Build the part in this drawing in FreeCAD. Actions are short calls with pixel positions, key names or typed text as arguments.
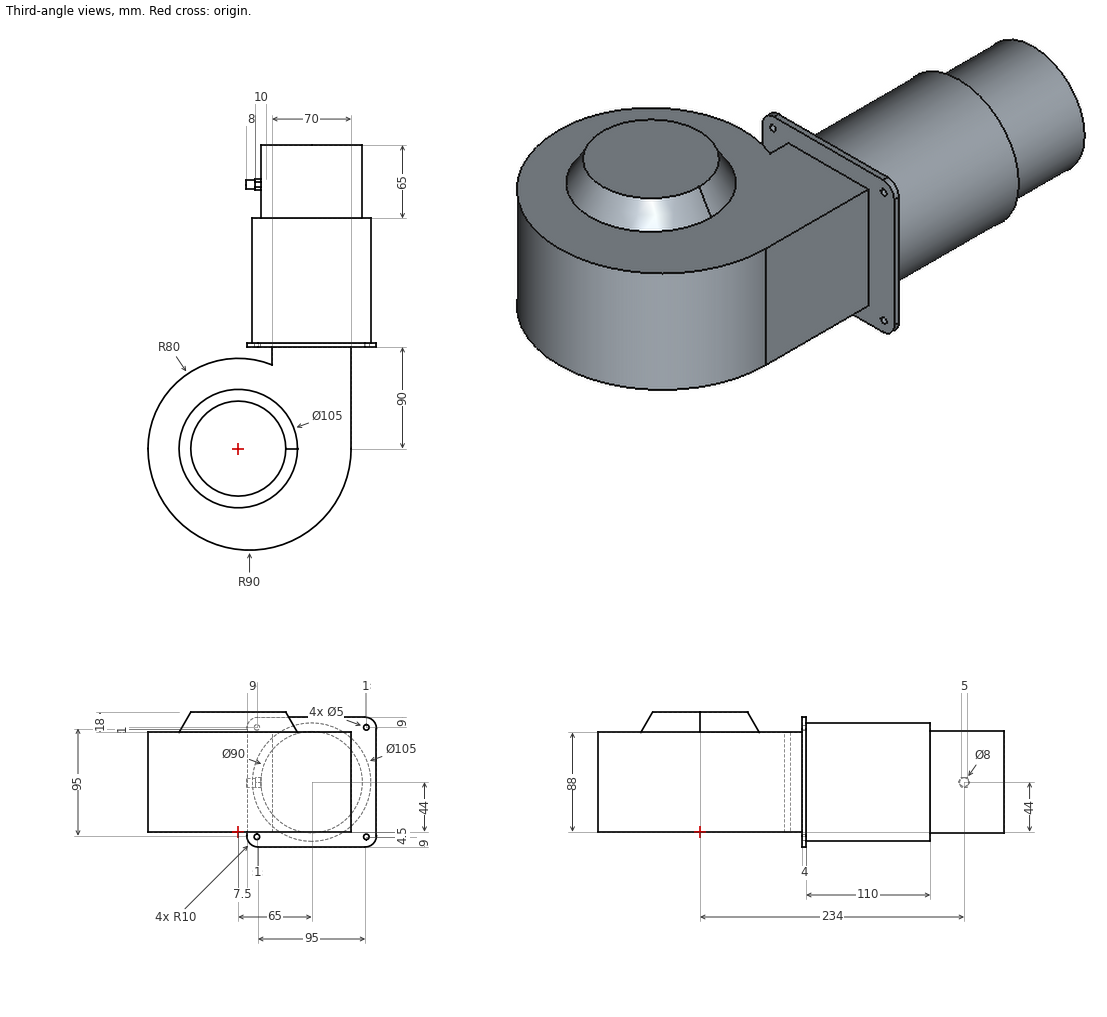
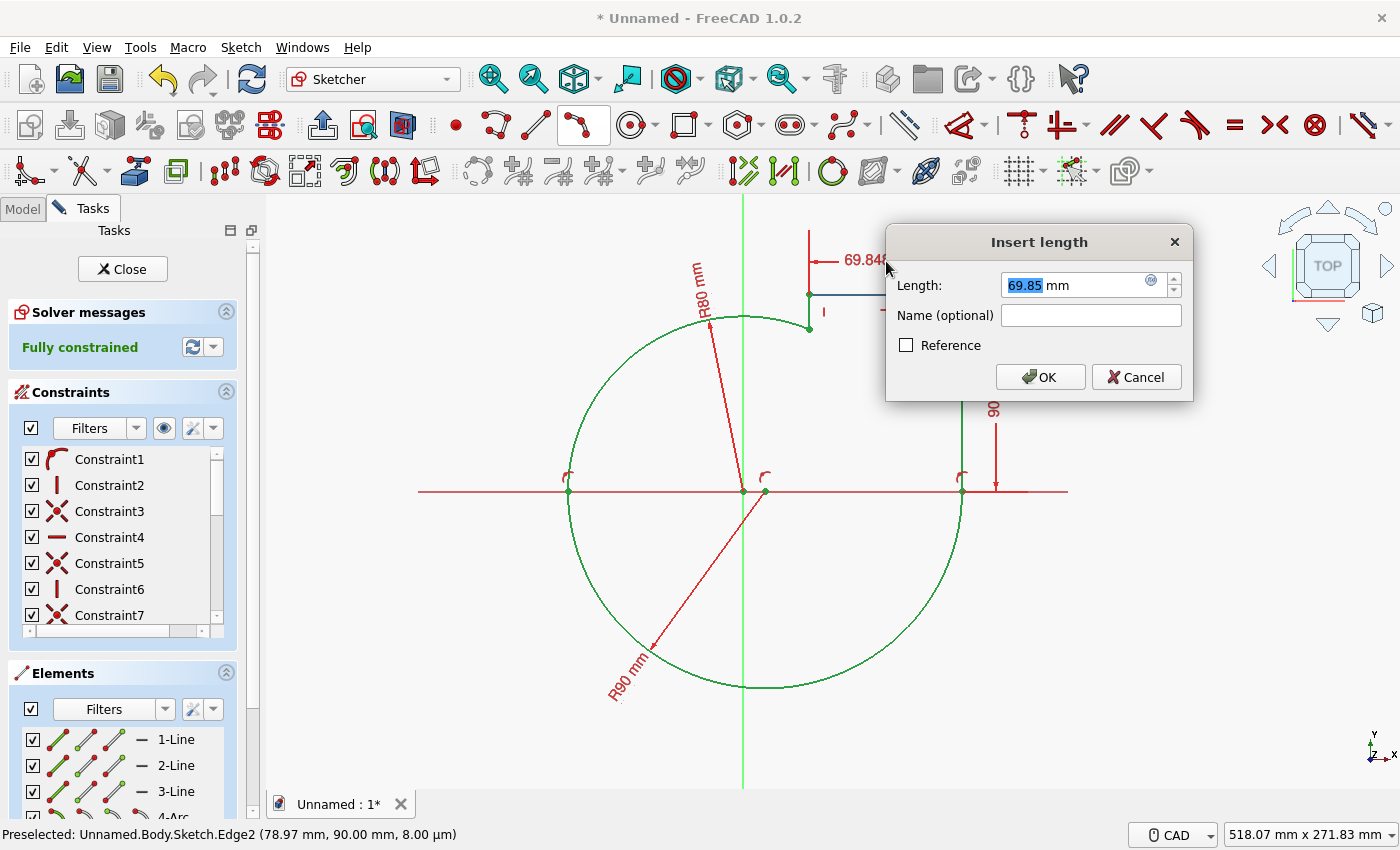
text(70)
key(Return)
key(Escape)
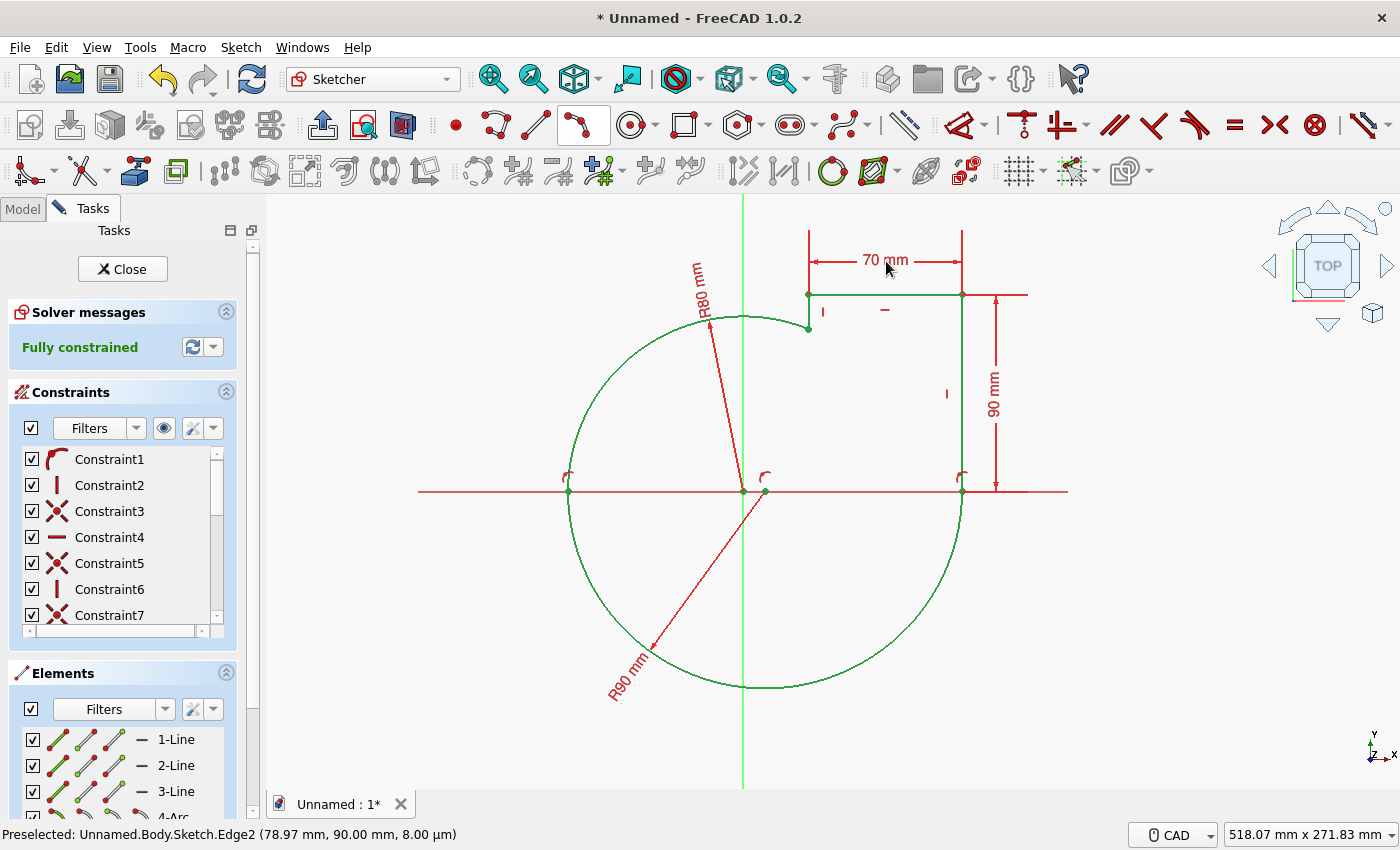
click(123, 269)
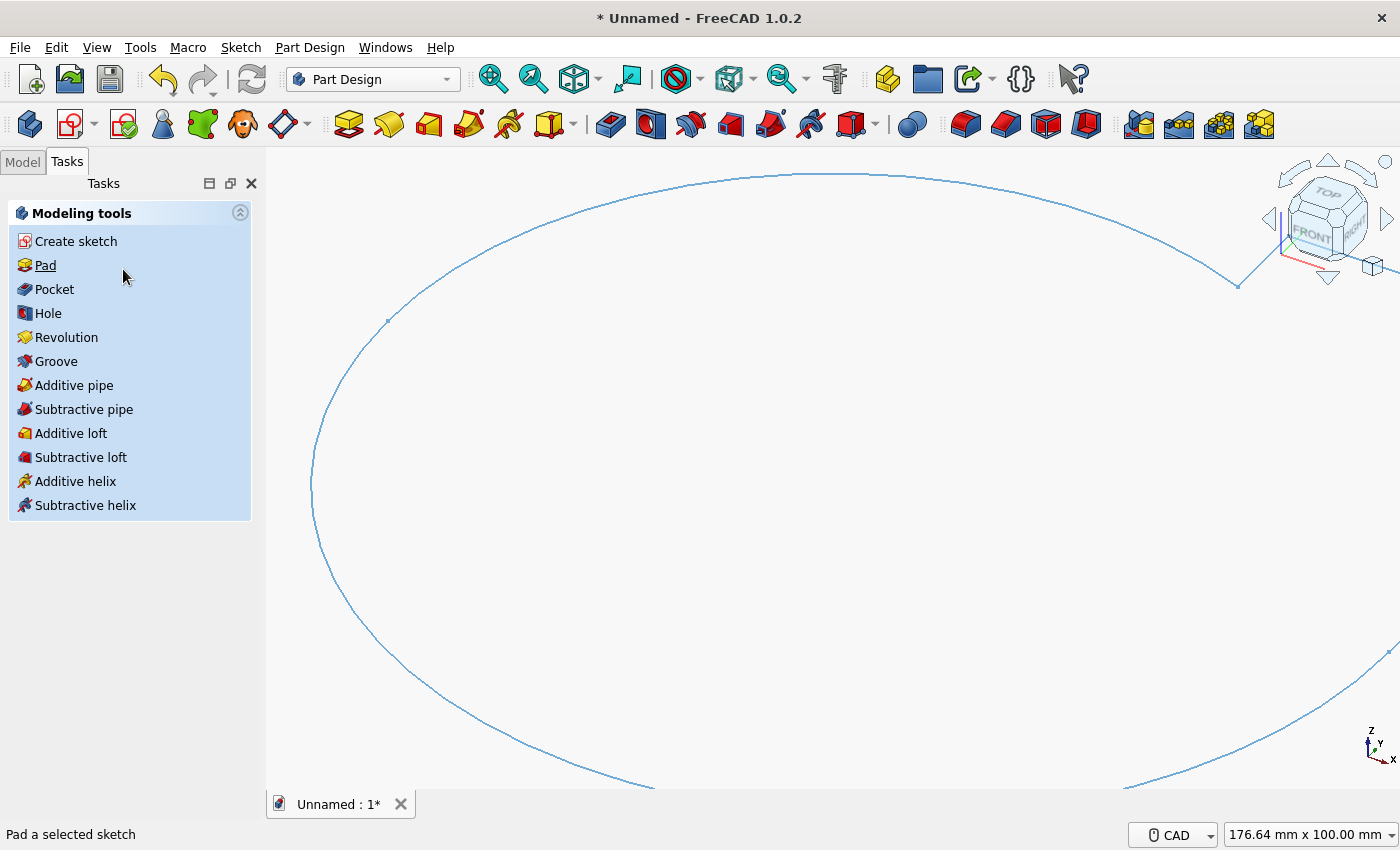
click(350, 124)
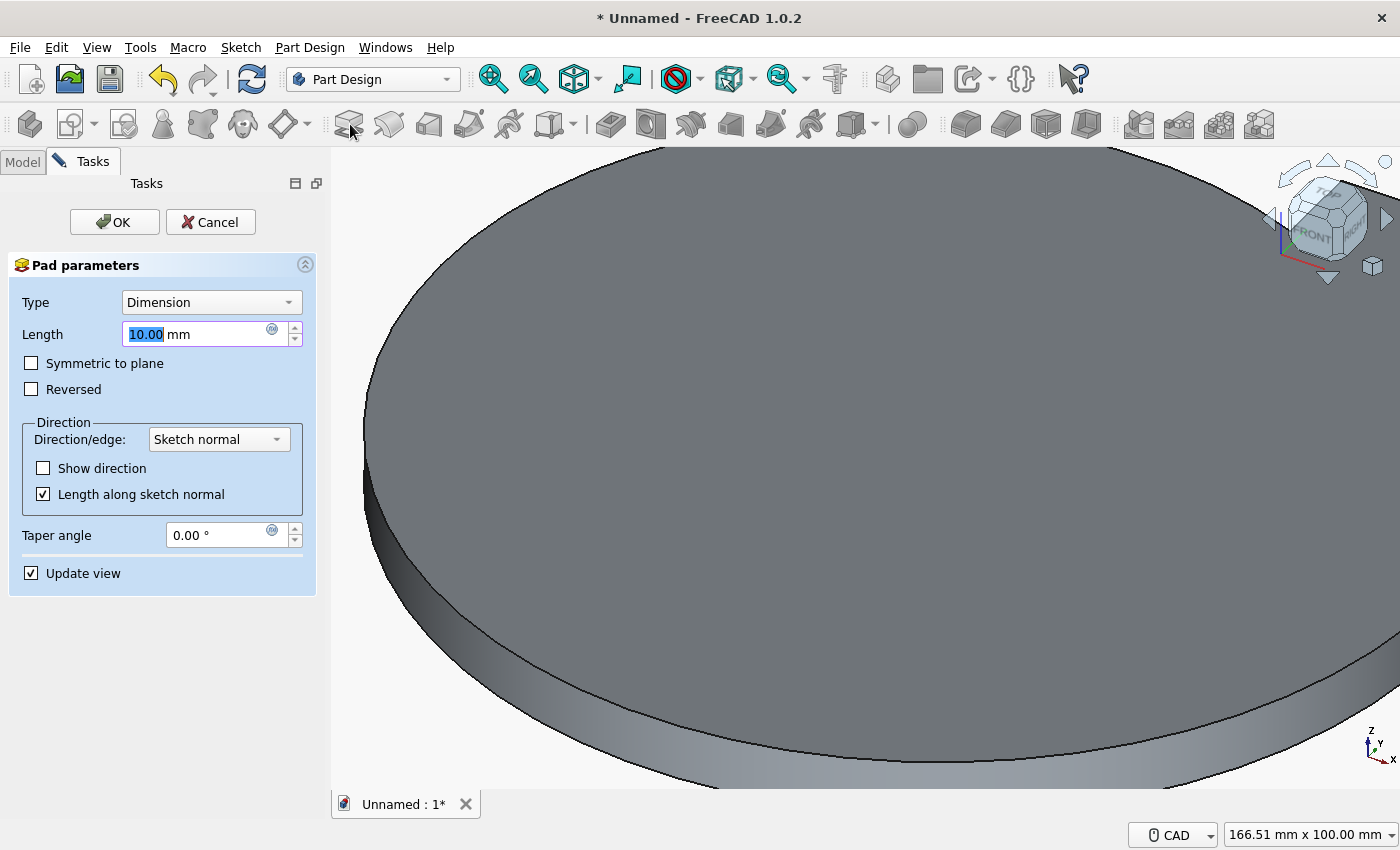
text(88)
key(Tab)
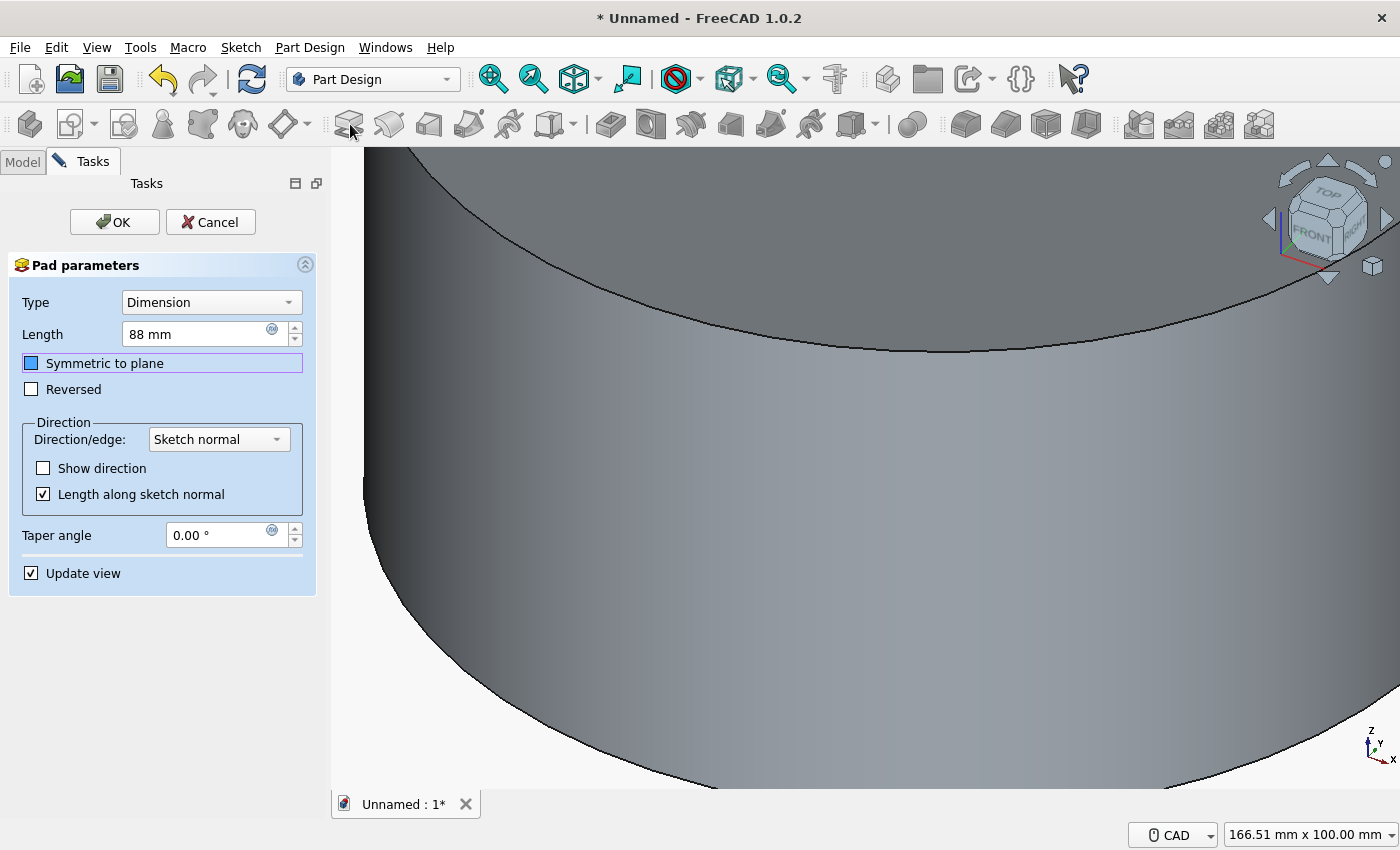
click(115, 222)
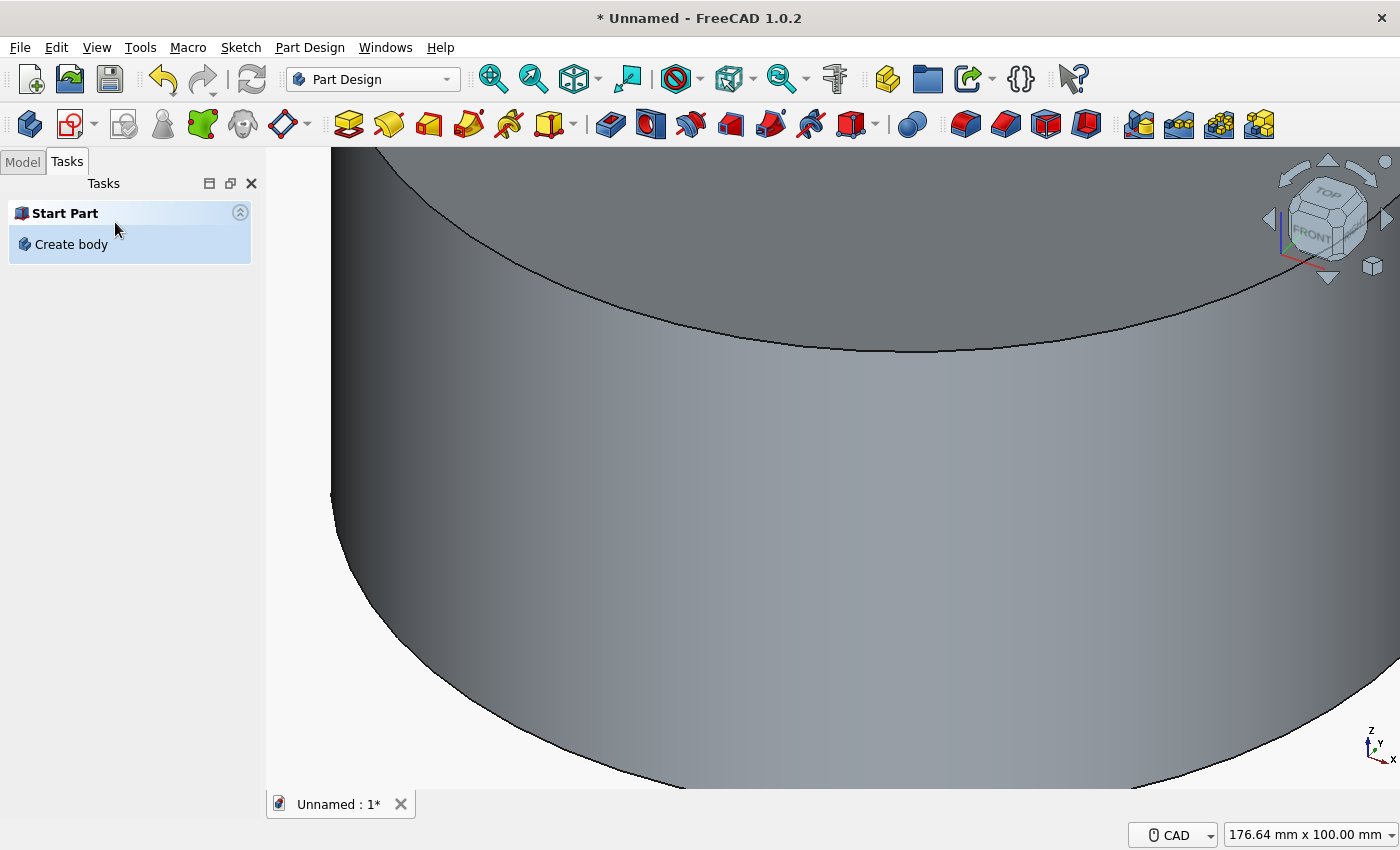
click(494, 80)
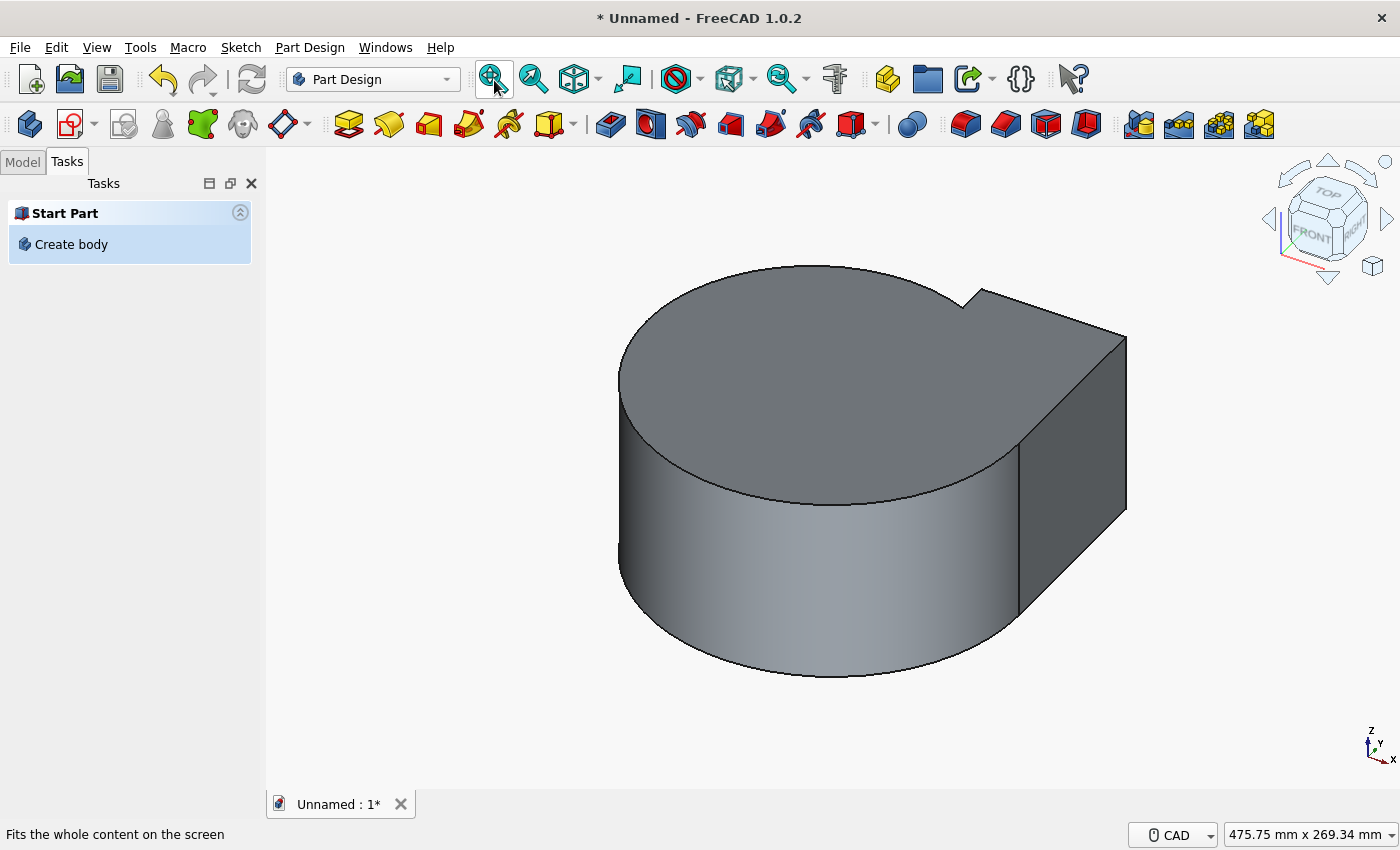
click(833, 381)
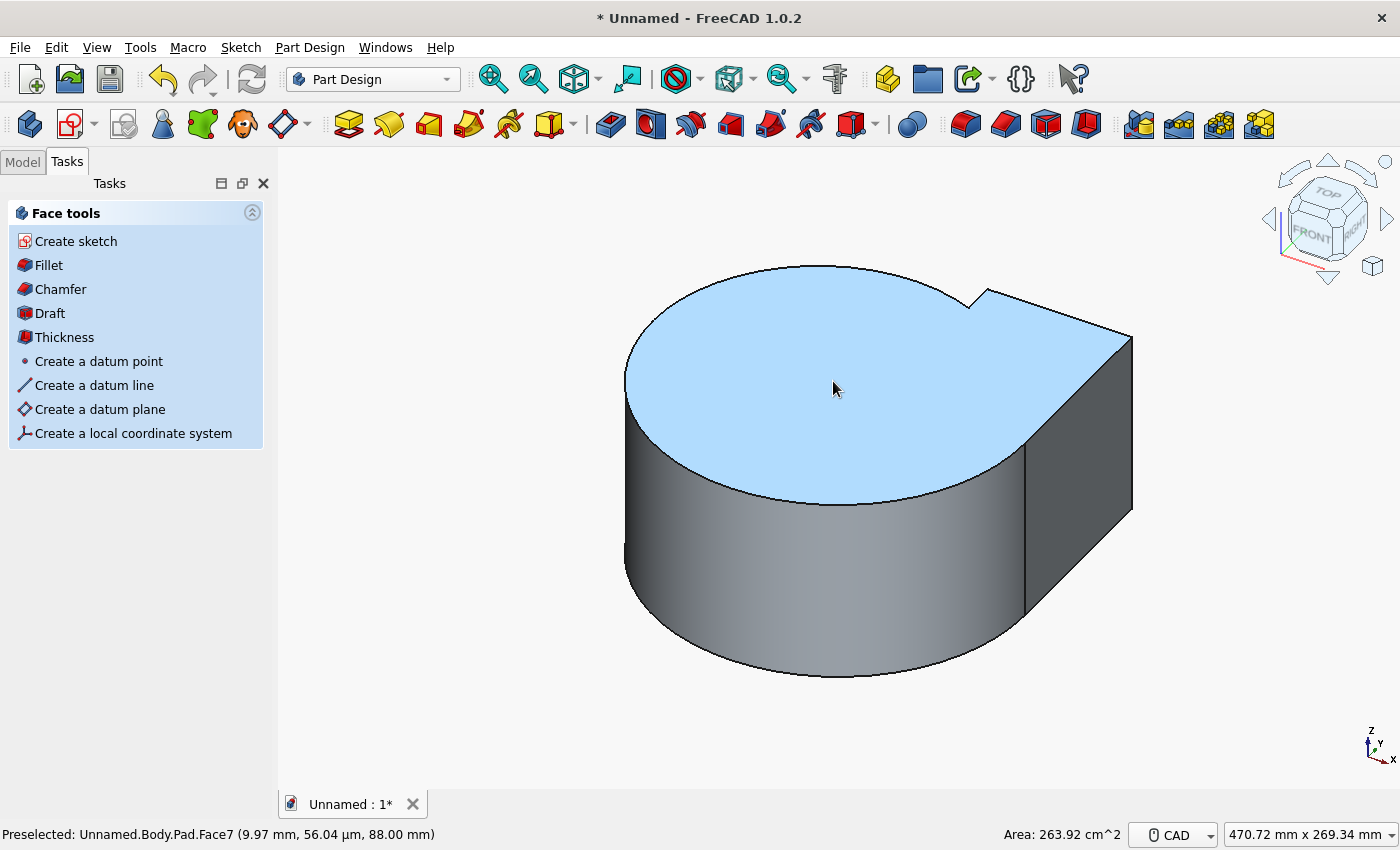
click(70, 124)